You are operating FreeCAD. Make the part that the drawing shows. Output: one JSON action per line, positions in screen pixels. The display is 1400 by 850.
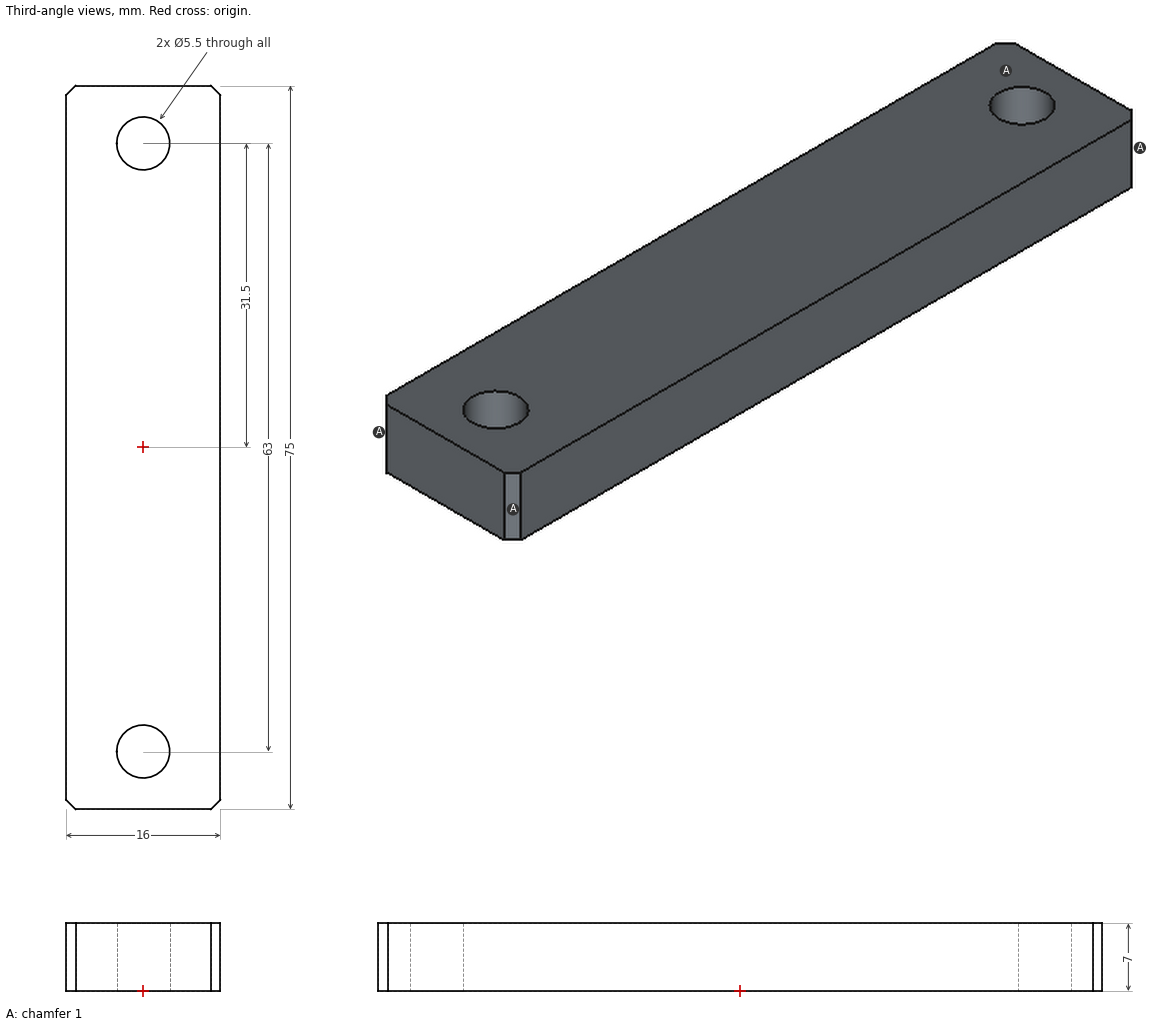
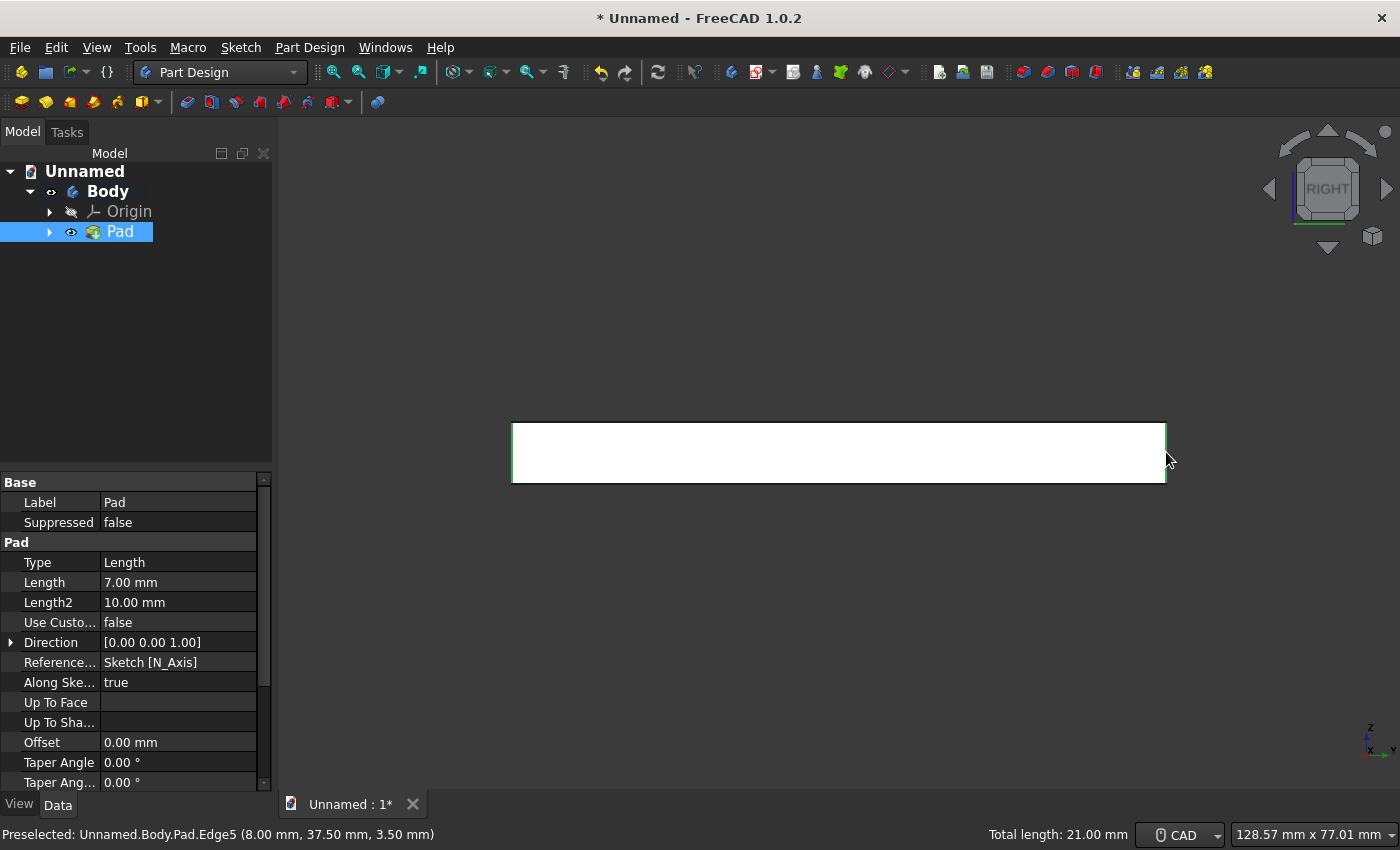
{"action": "key", "text": "5"}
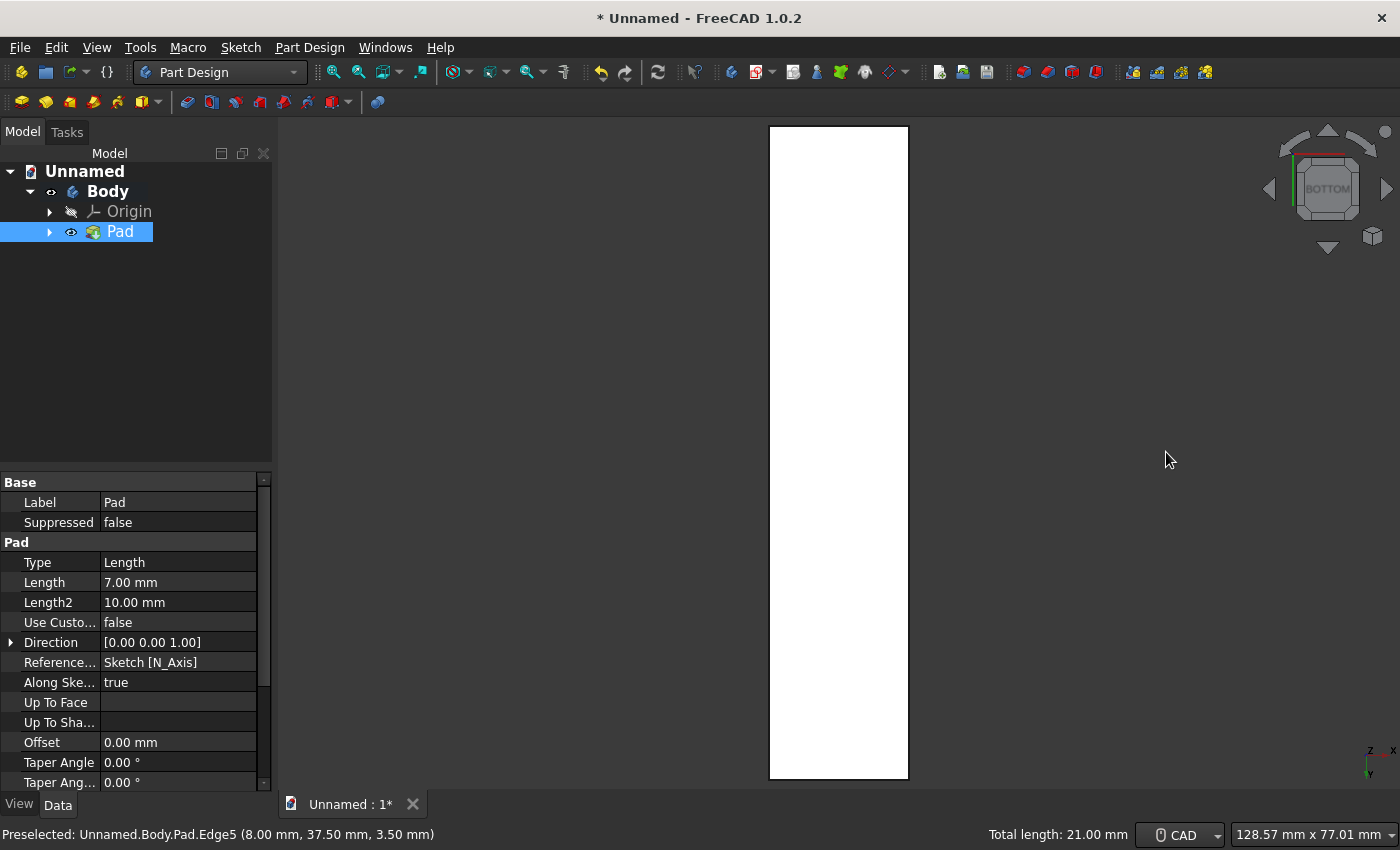
{"action": "key", "text": "4"}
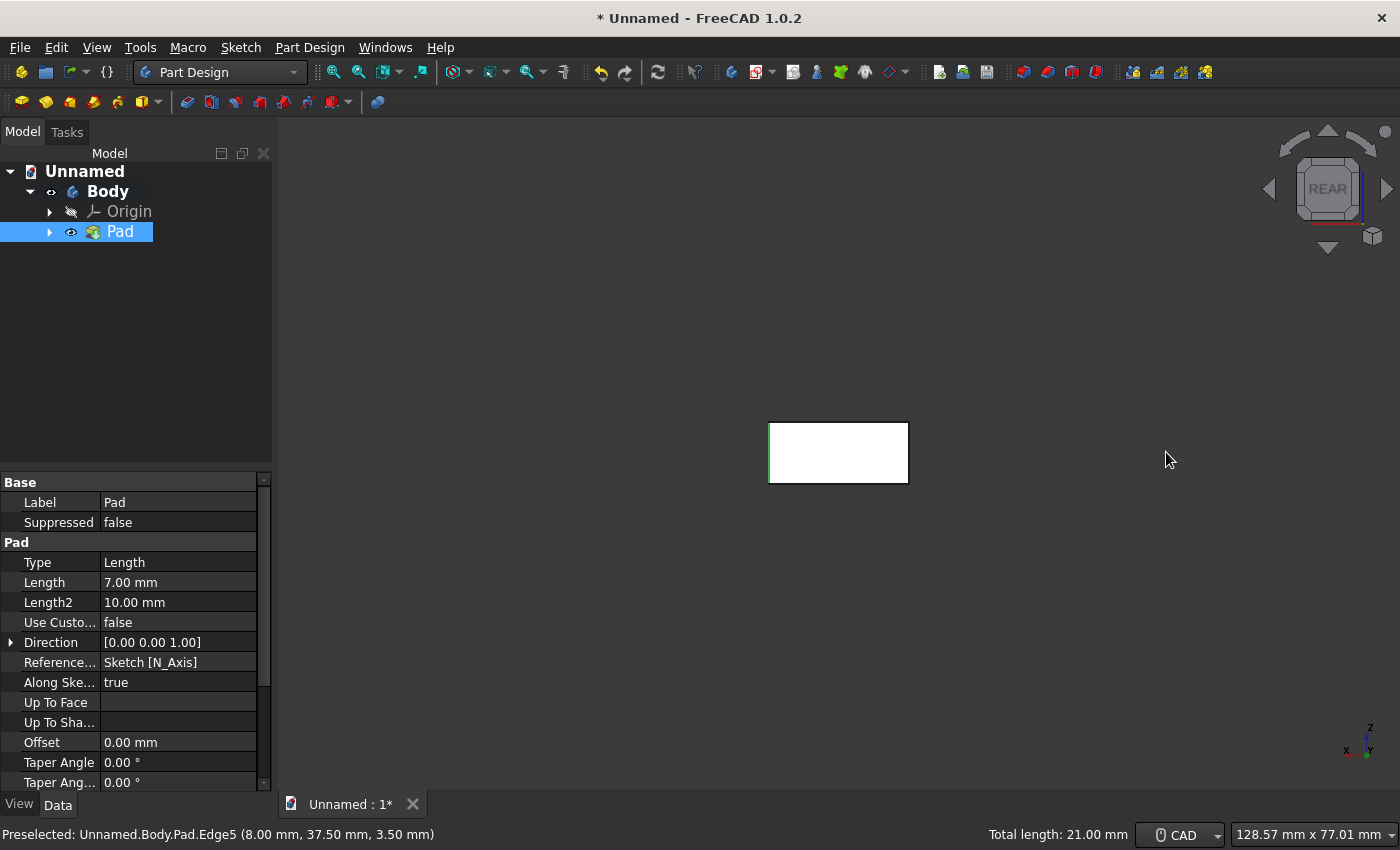
{"action": "left_click", "coordinate": [334, 72]}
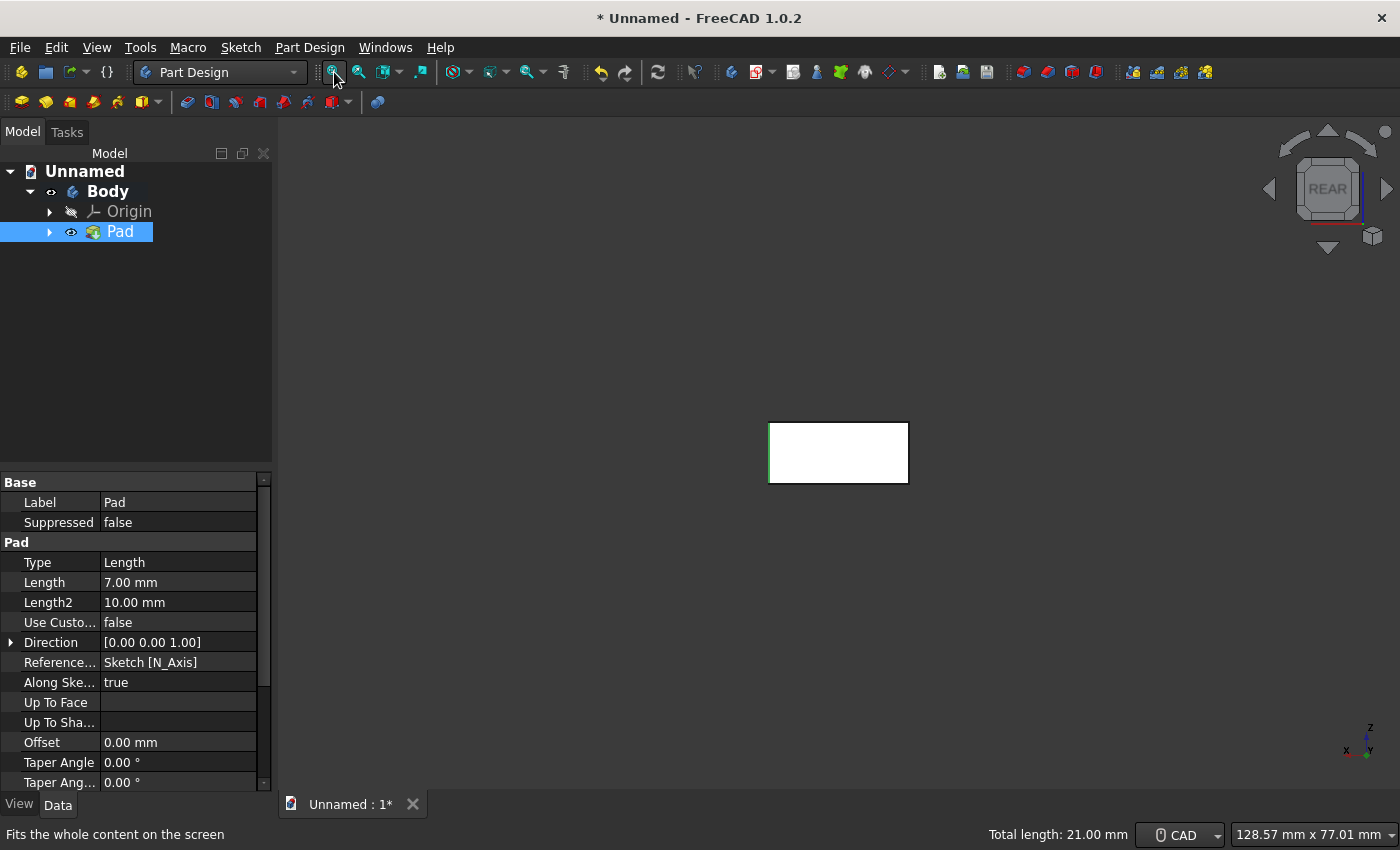
{"action": "left_click", "coordinate": [909, 452], "text": "ctrl"}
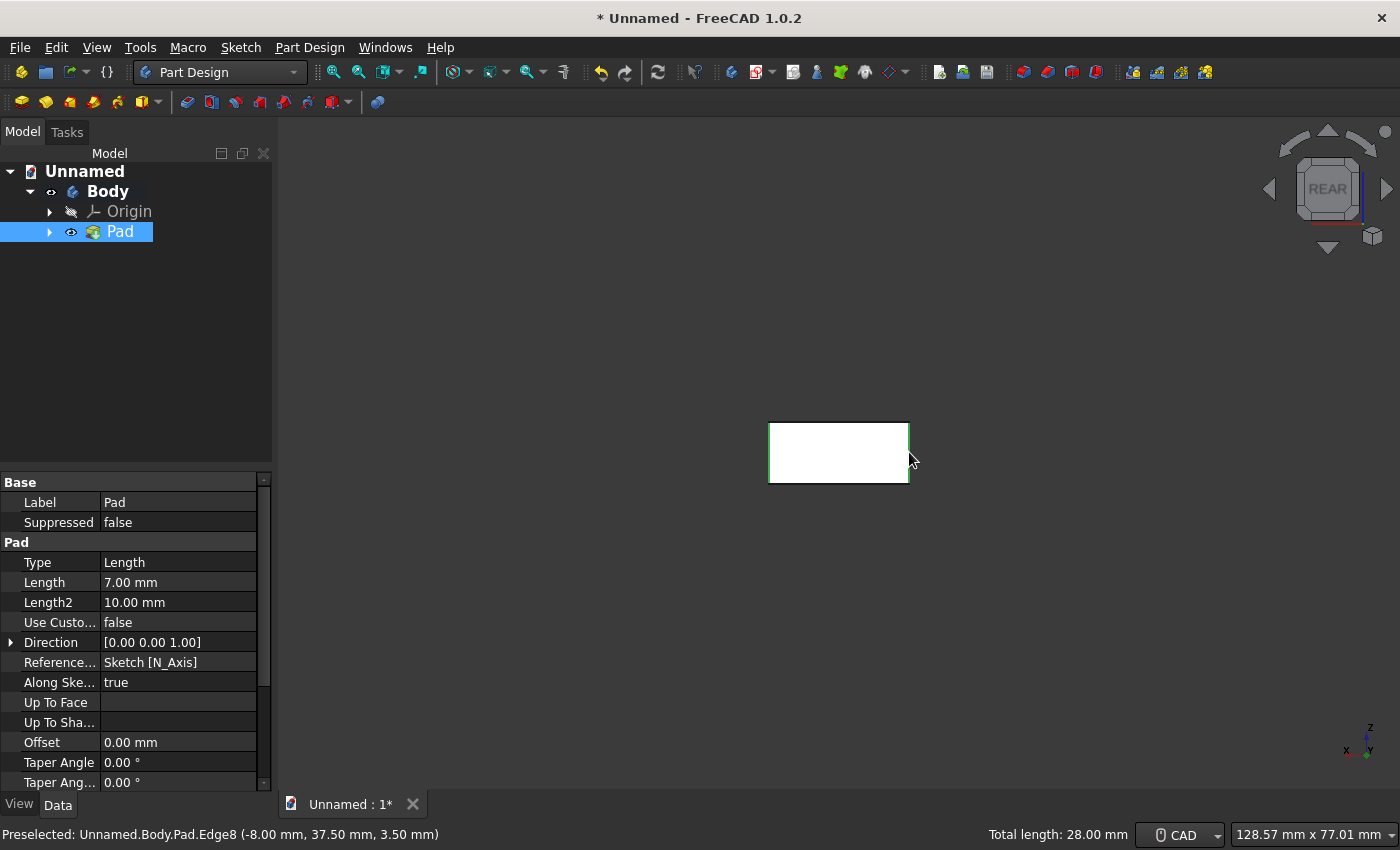
{"action": "left_click", "coordinate": [1048, 72]}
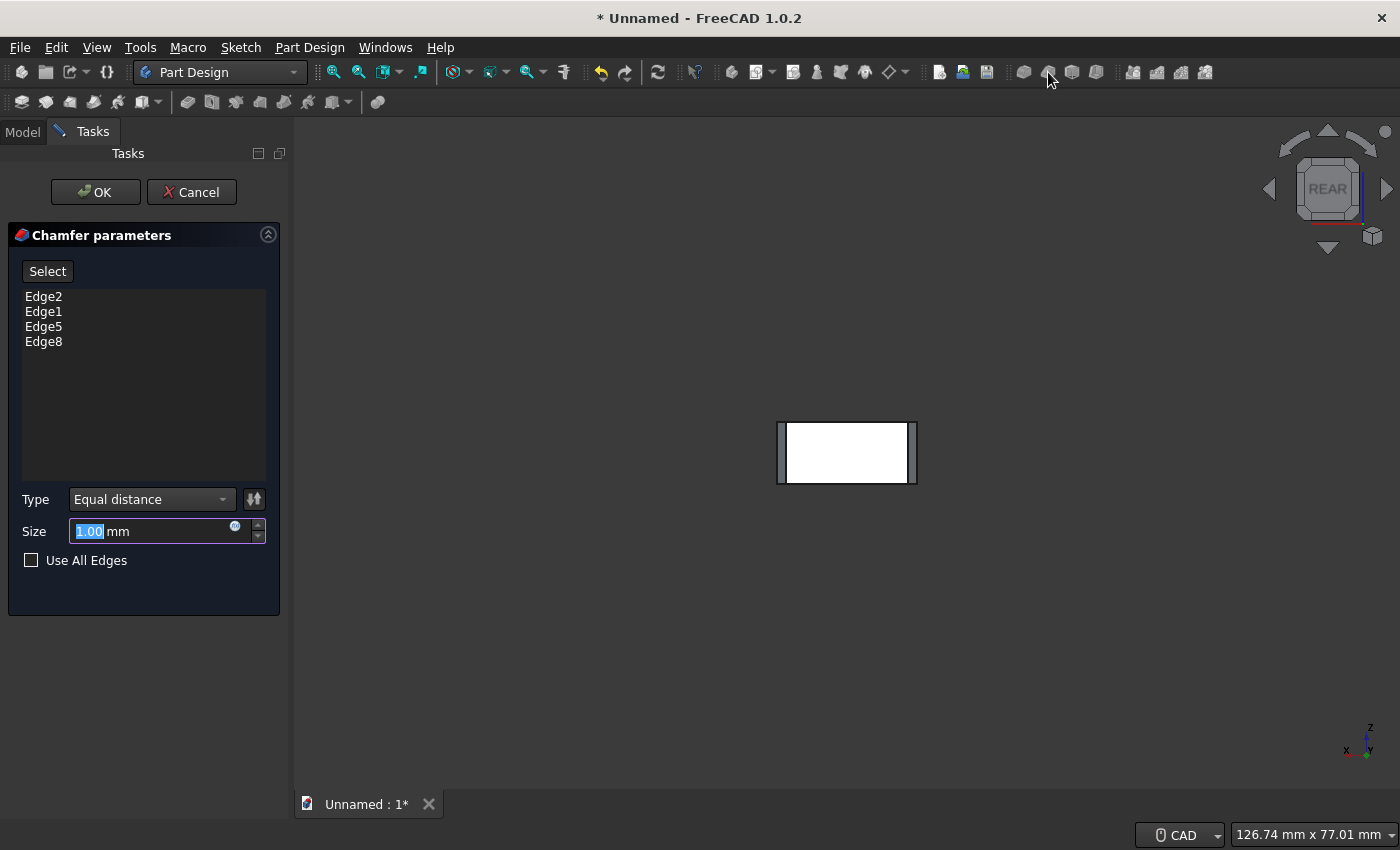
{"action": "type", "text": "1"}
{"action": "key", "text": "Tab"}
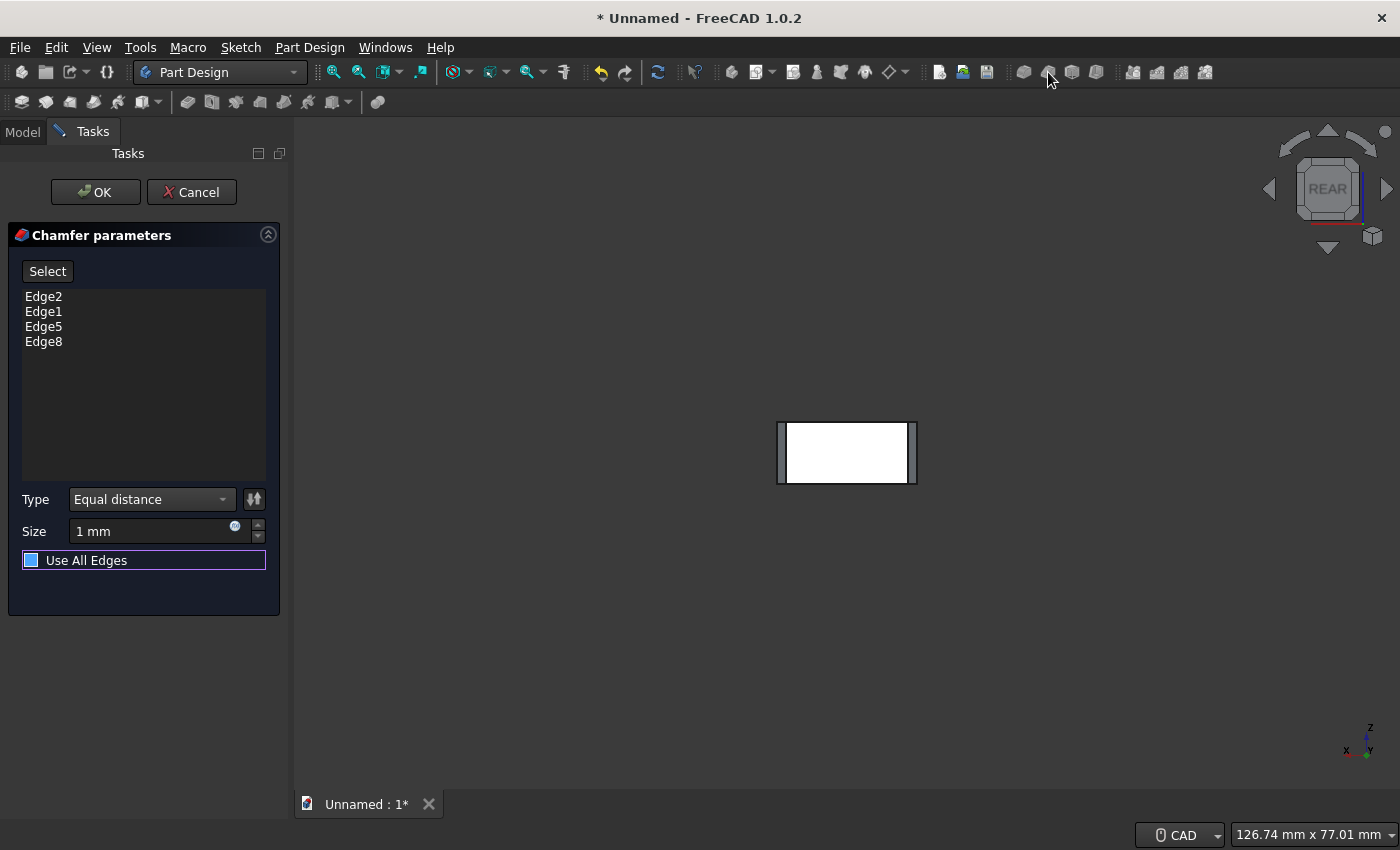
{"action": "left_click", "coordinate": [96, 192]}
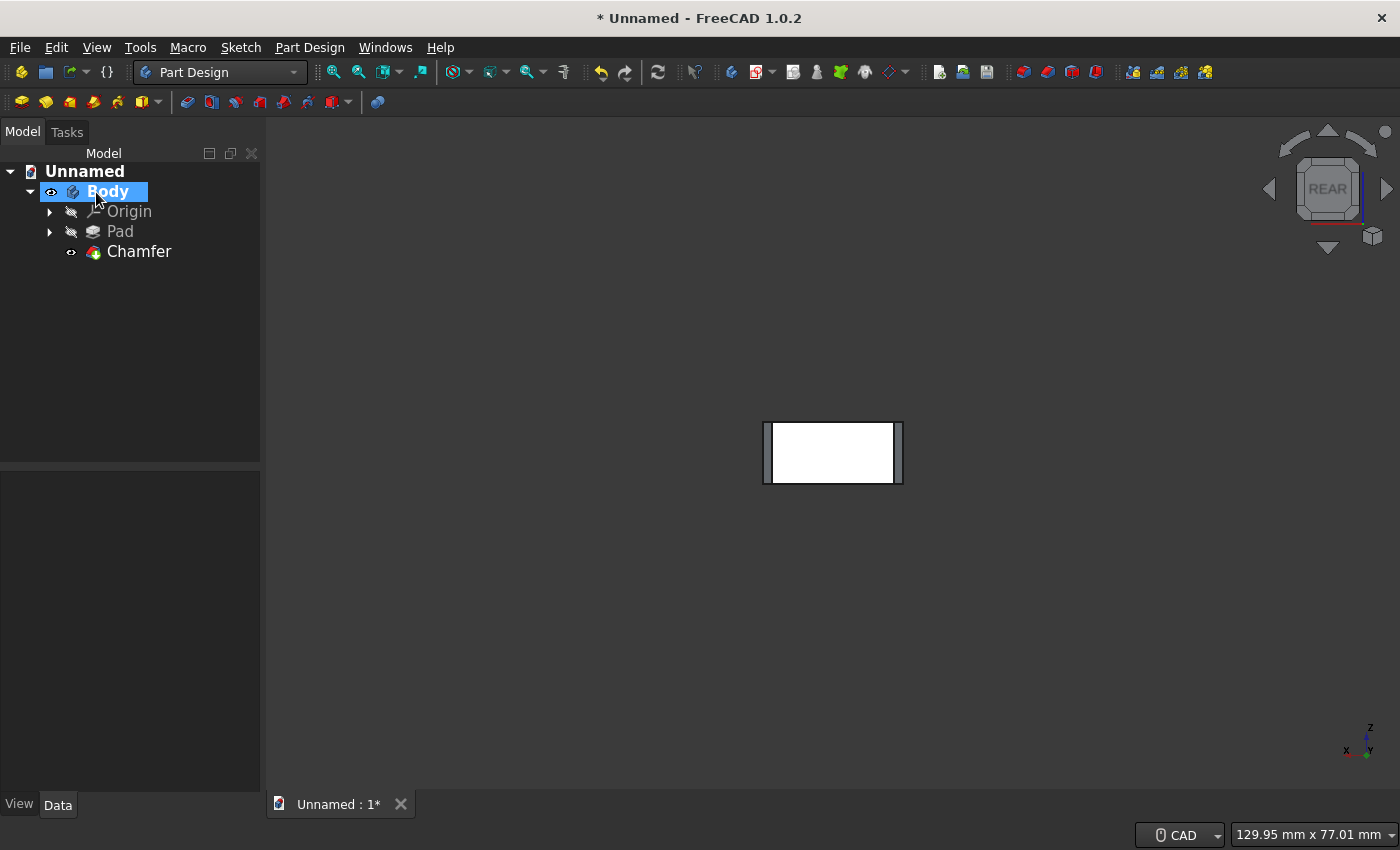
{"action": "left_click", "coordinate": [334, 72]}